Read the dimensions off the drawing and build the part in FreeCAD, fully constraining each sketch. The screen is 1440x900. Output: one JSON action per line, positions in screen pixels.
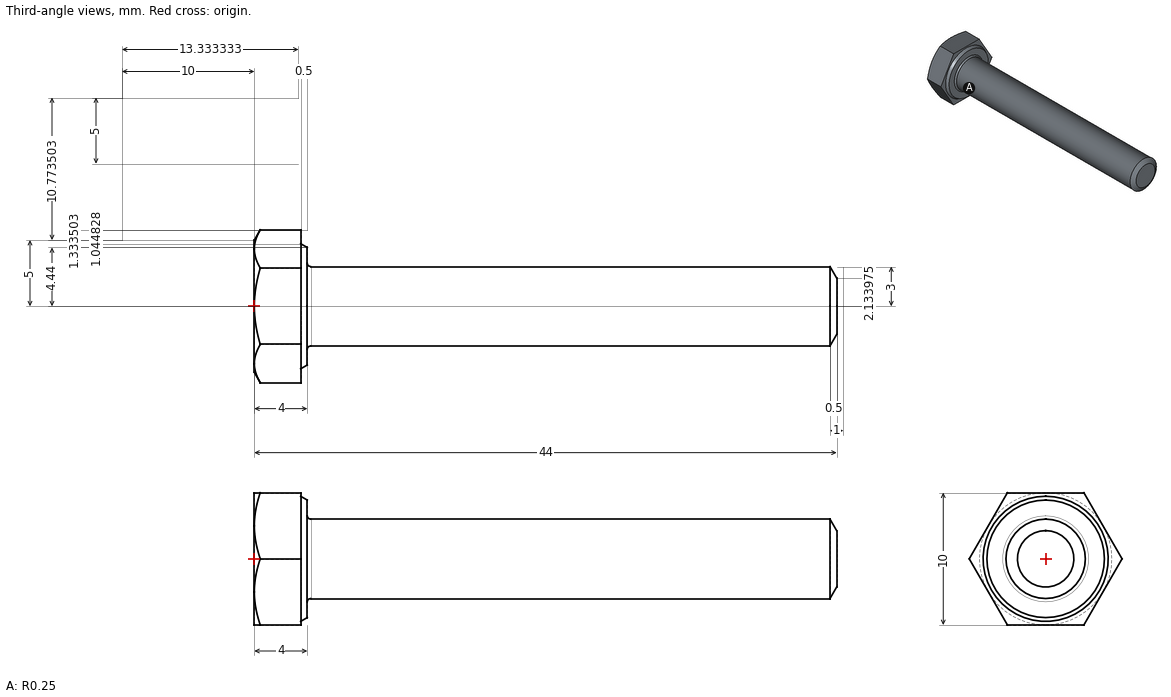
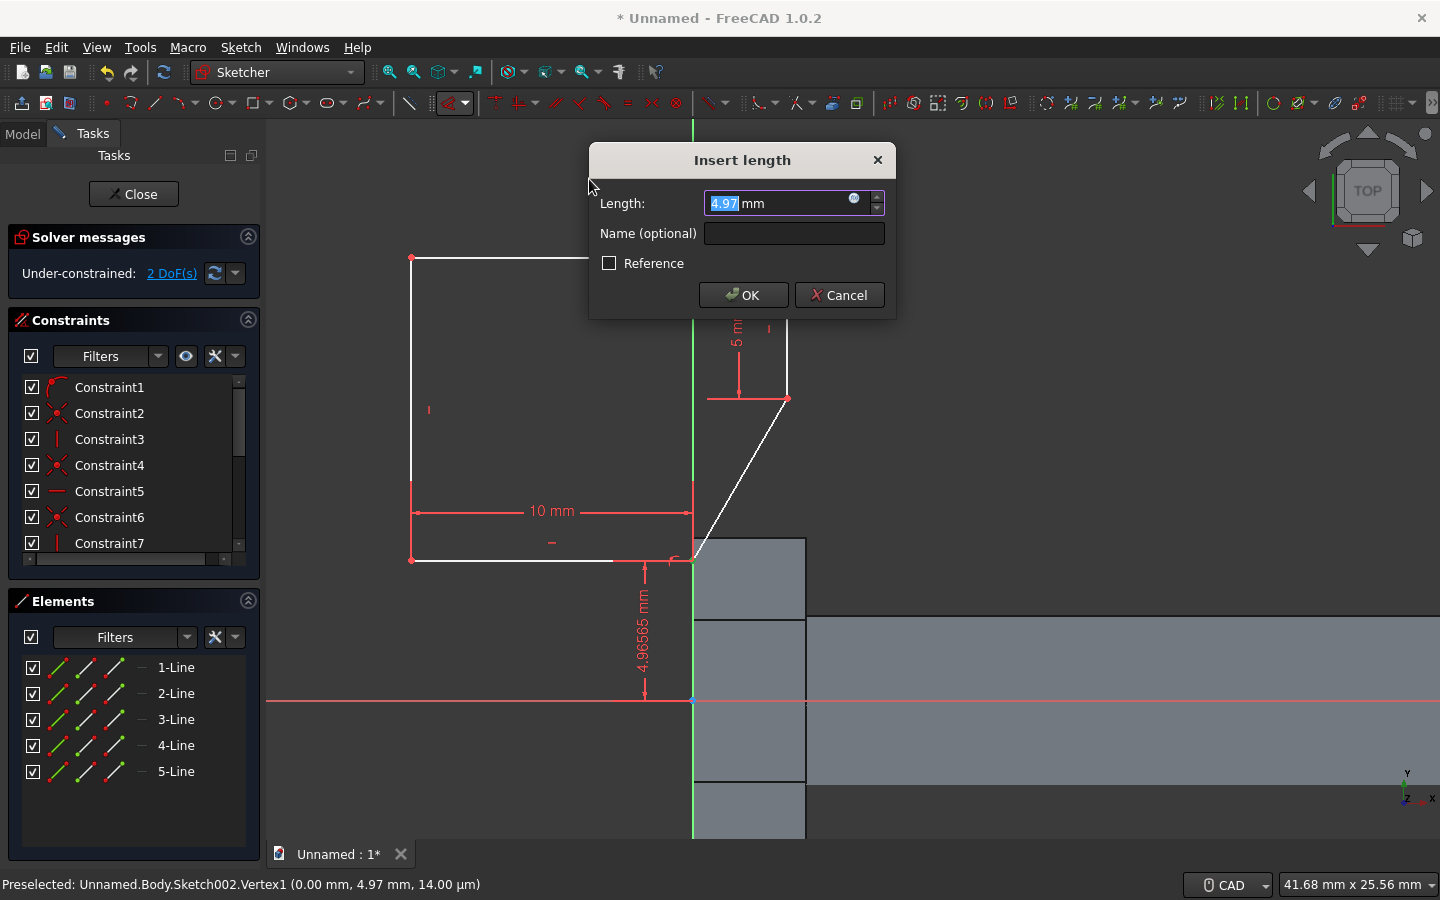
{"action": "type", "text": "5"}
{"action": "key", "text": "Return"}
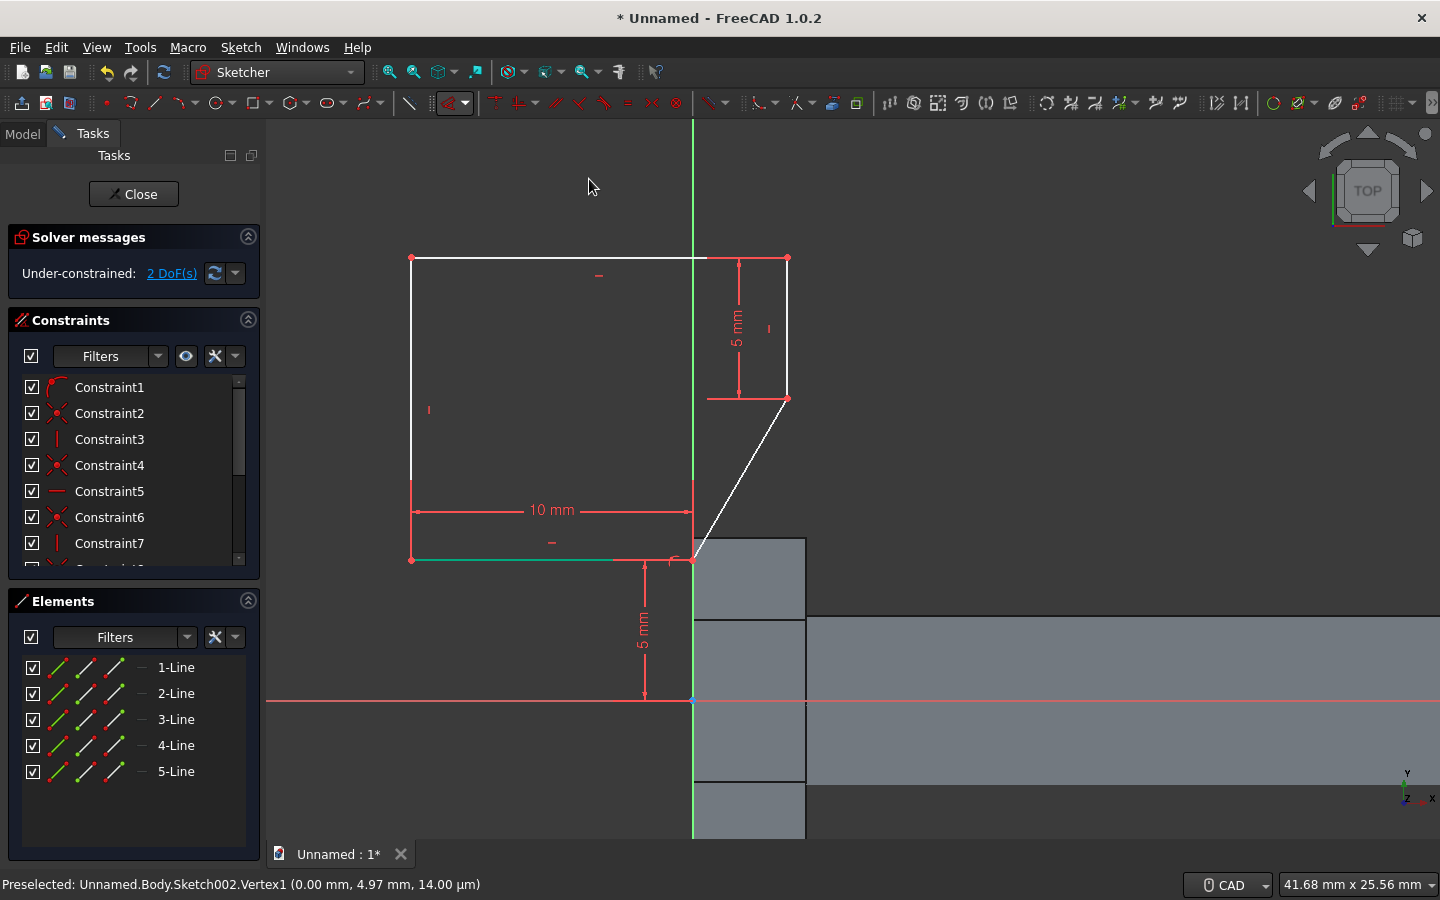
{"action": "left_click", "coordinate": [674, 258]}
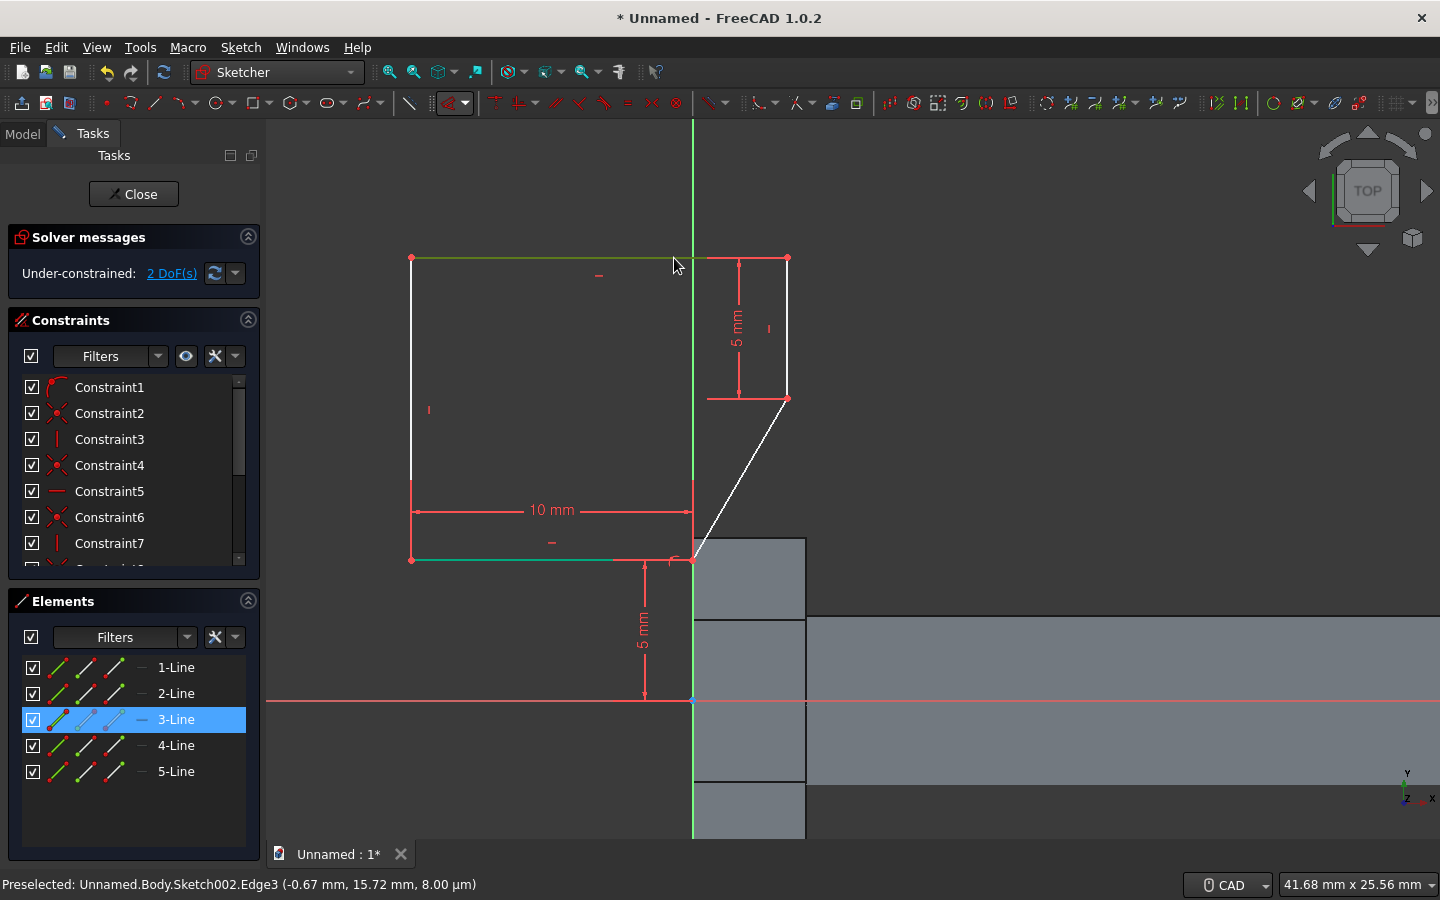
{"action": "key", "text": "l"}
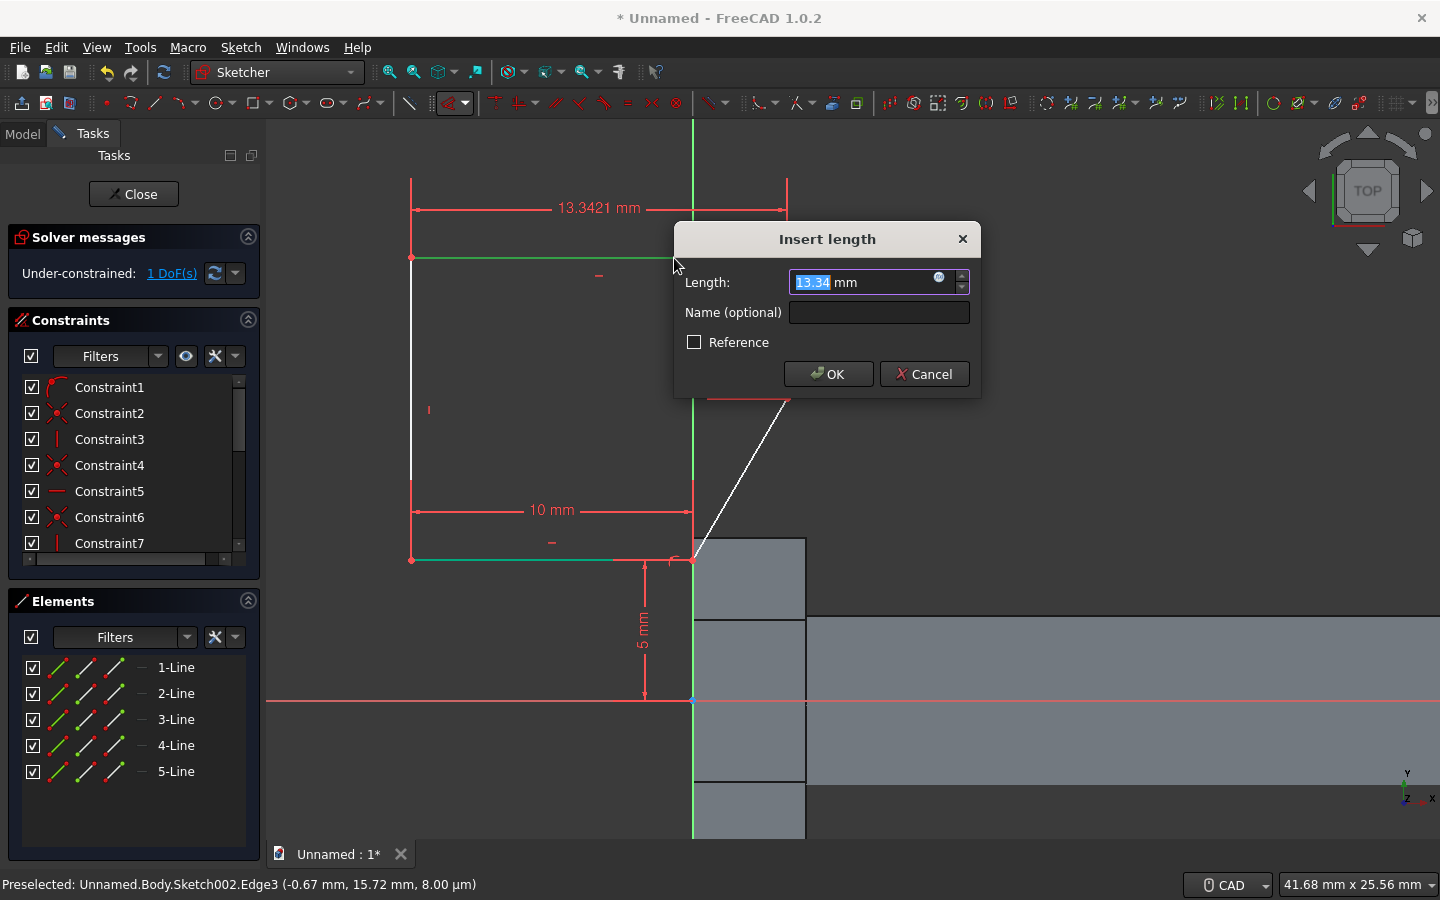
{"action": "type", "text": "13.333333"}
{"action": "key", "text": "Return"}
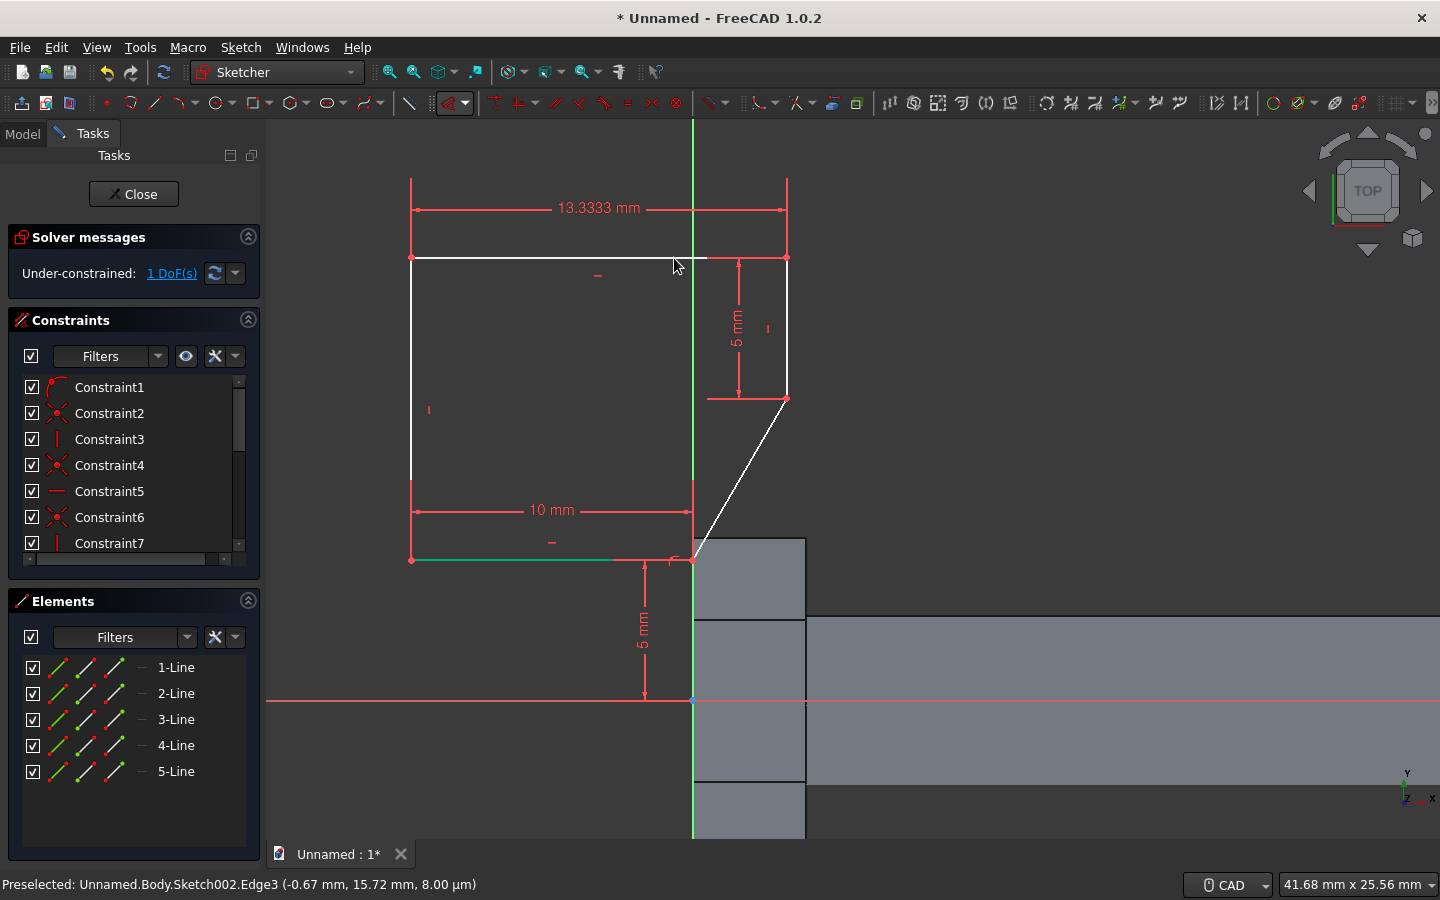
{"action": "left_click", "coordinate": [411, 349]}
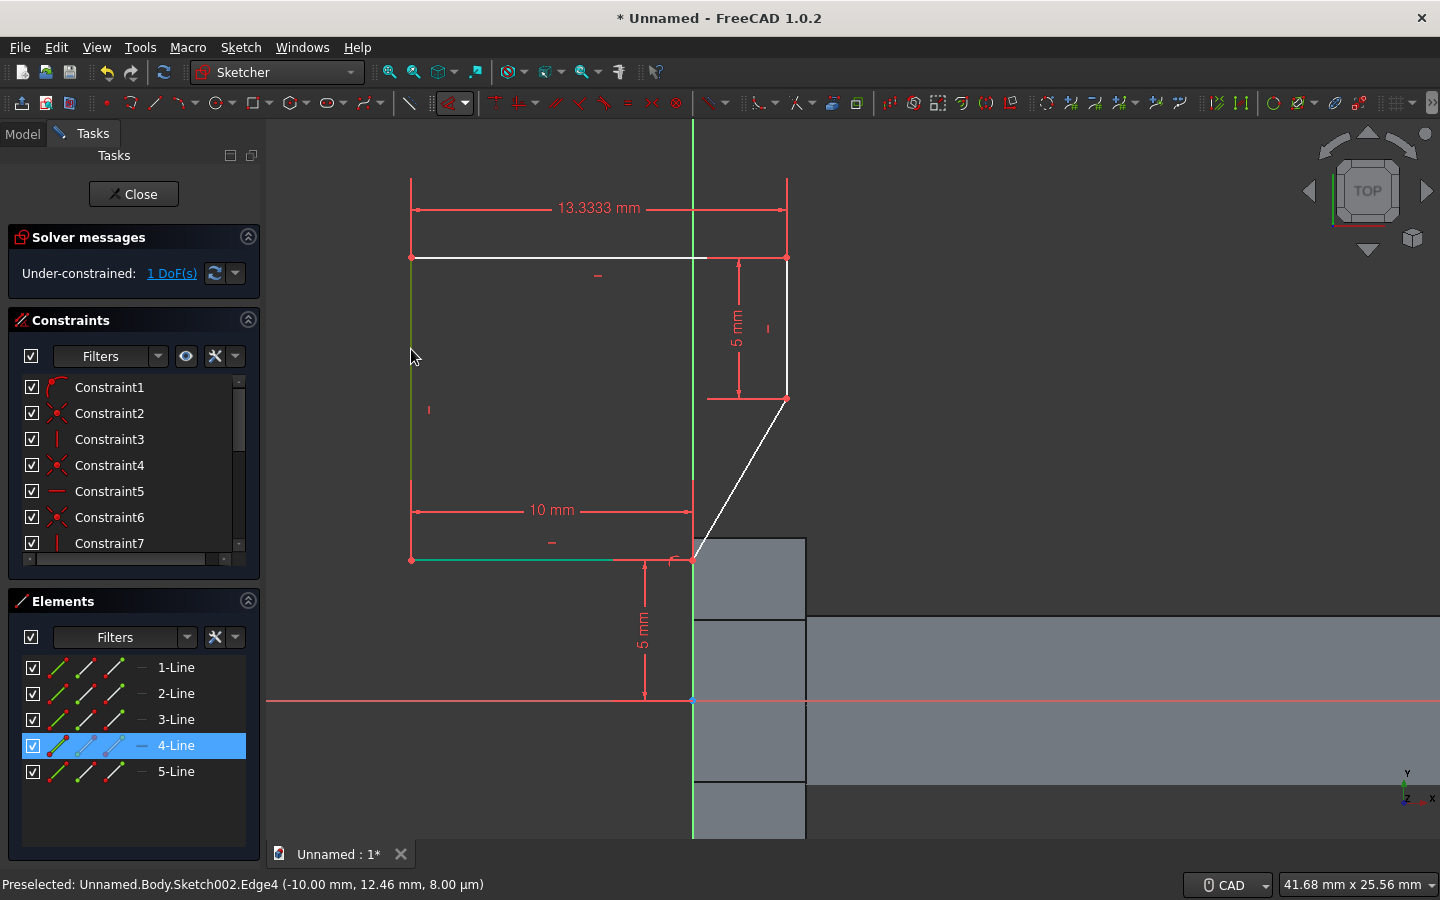
{"action": "key", "text": "i"}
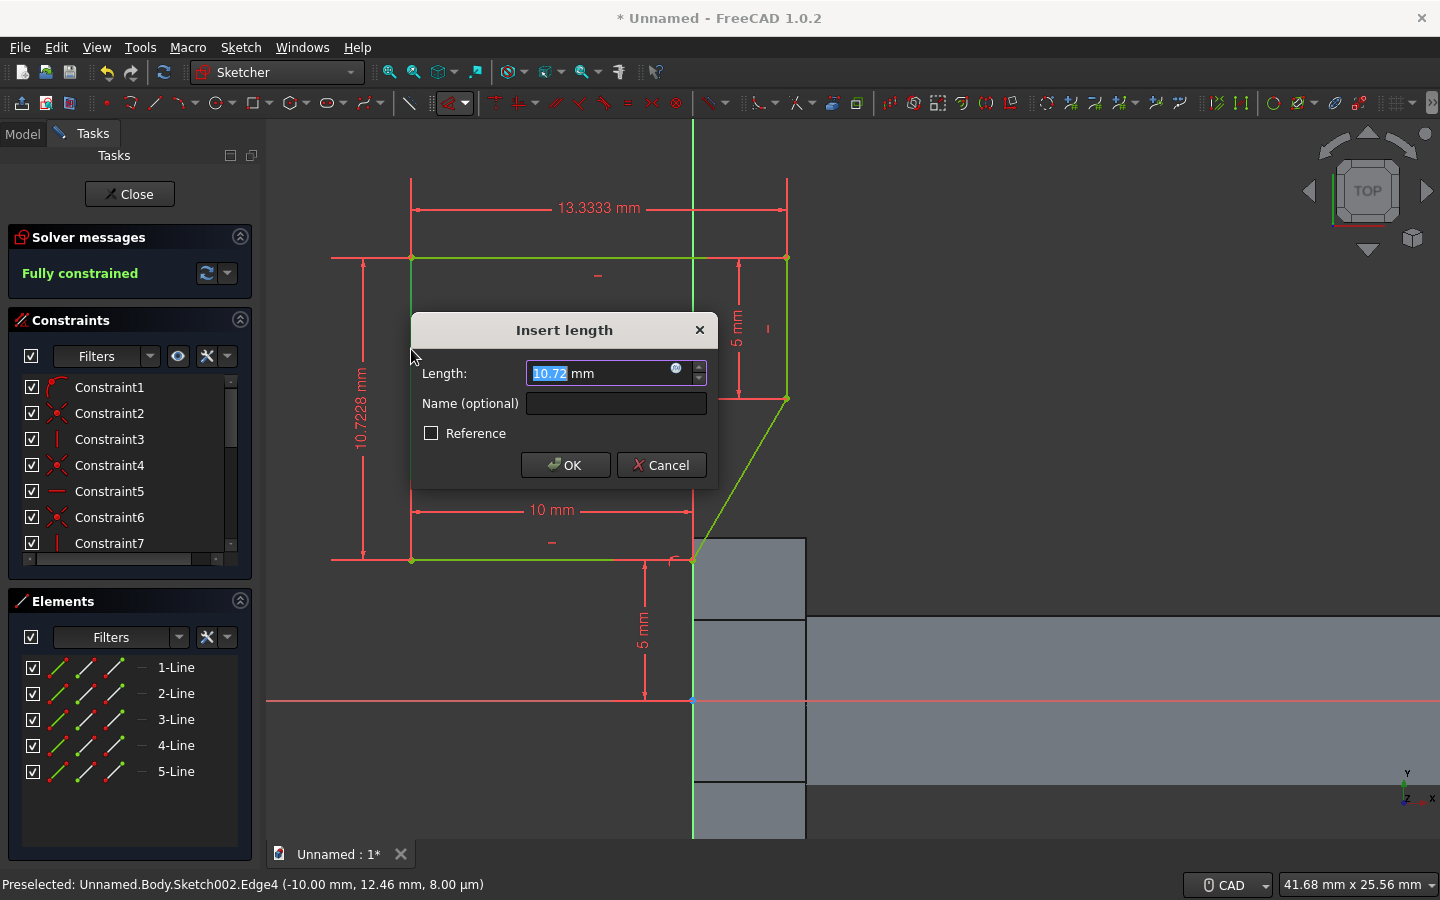
{"action": "type", "text": "10.773503"}
{"action": "key", "text": "Return"}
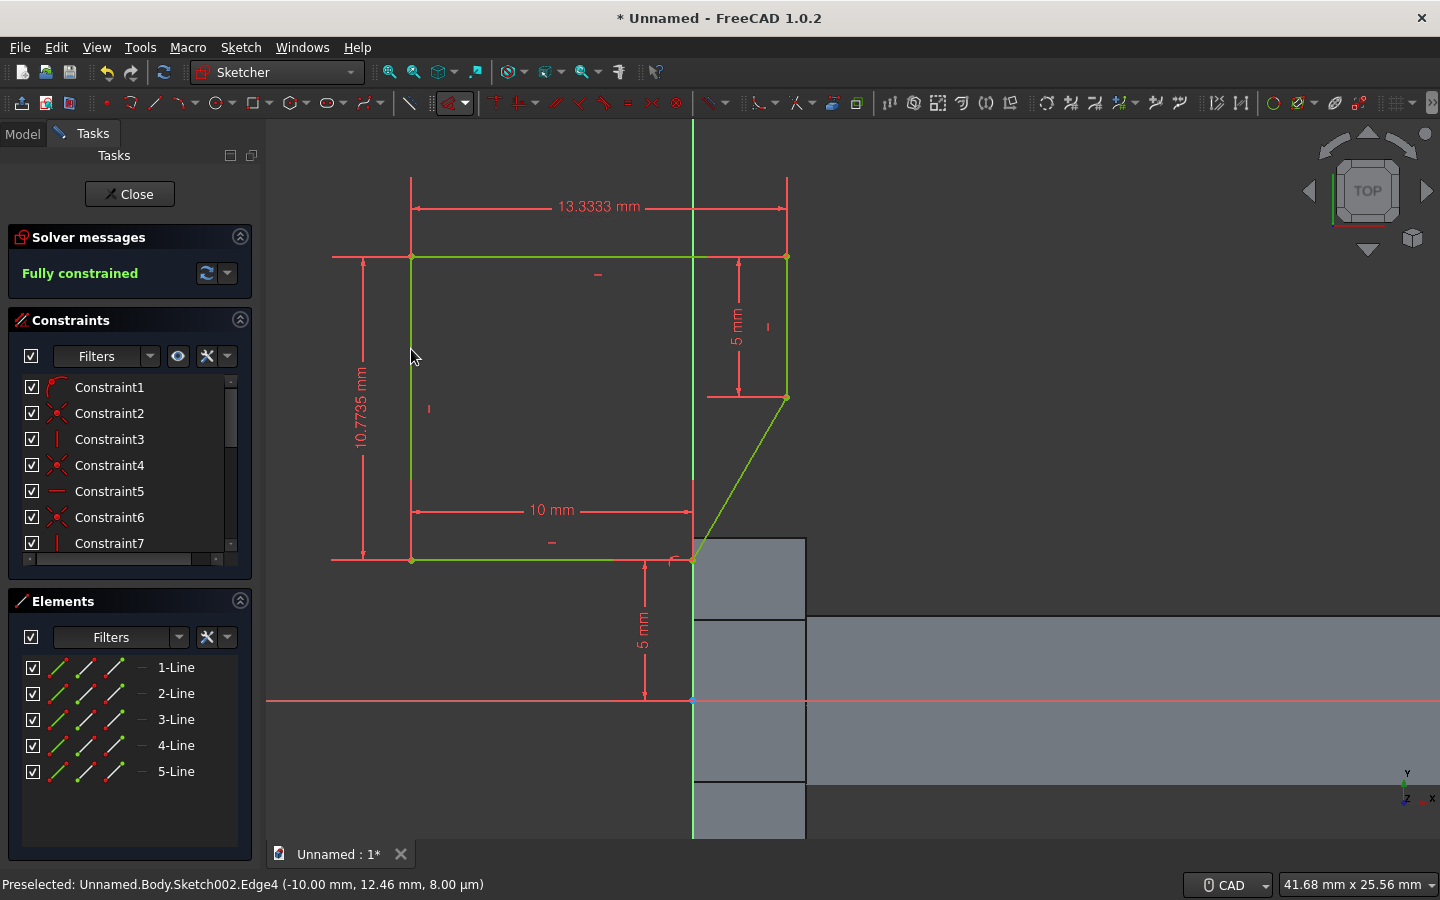
{"action": "left_click", "coordinate": [130, 194]}